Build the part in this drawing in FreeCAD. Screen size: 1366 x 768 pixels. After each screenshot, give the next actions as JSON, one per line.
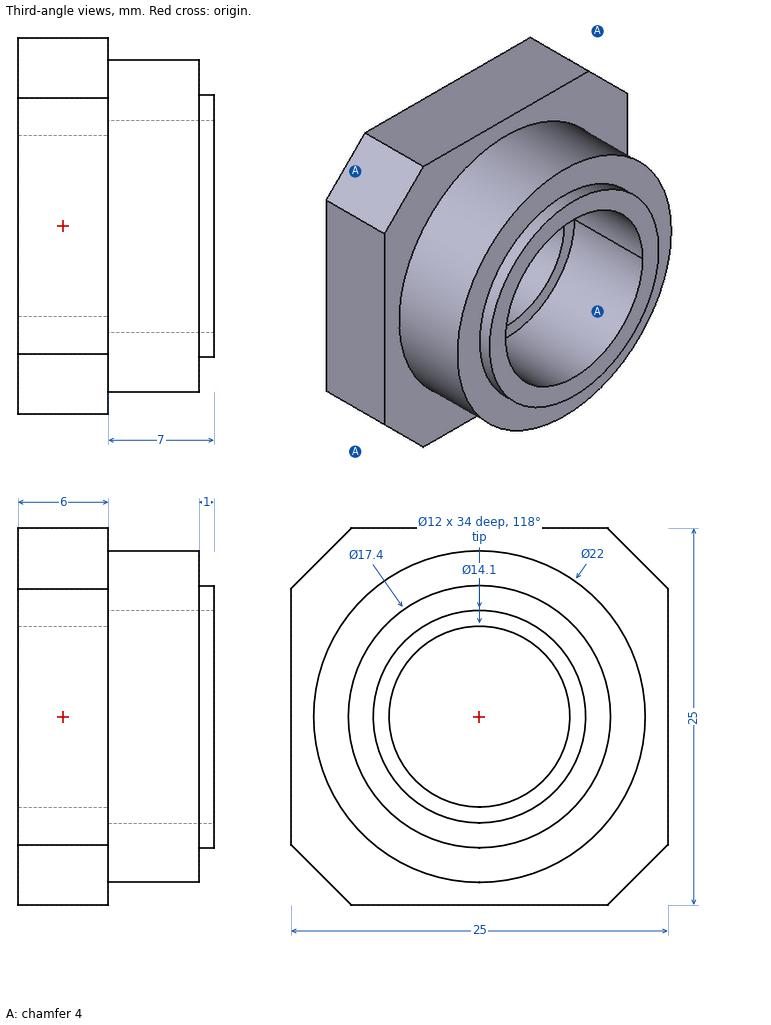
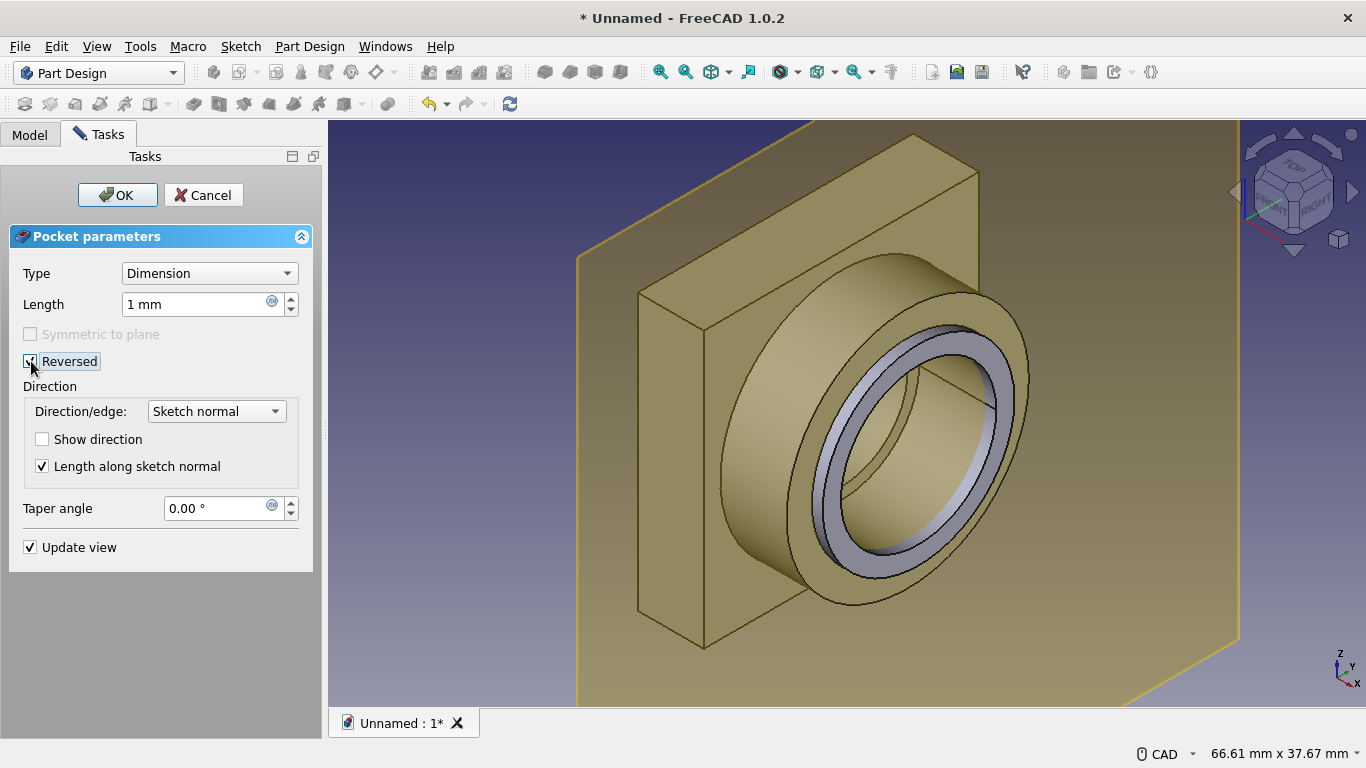
{"action": "left_click", "coordinate": [118, 195]}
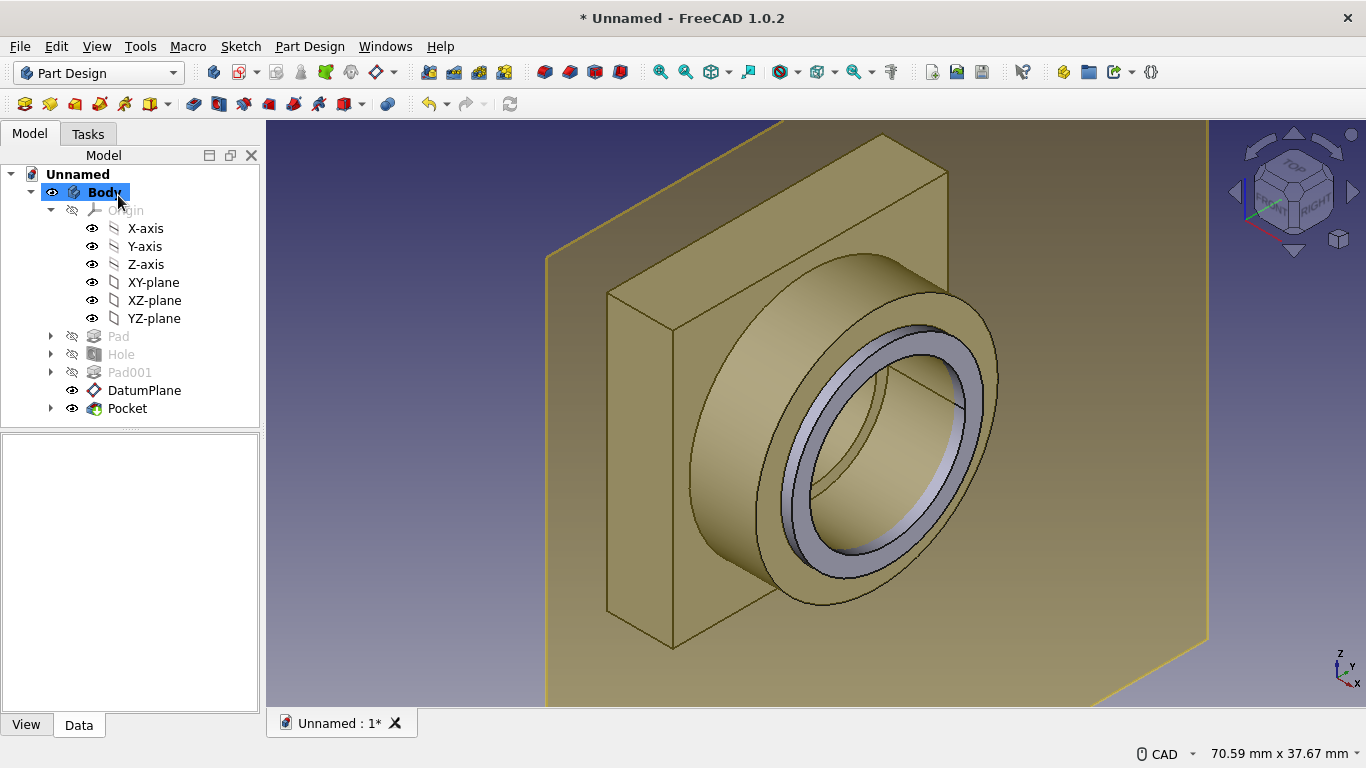
{"action": "left_click", "coordinate": [117, 390]}
{"action": "key", "text": "space"}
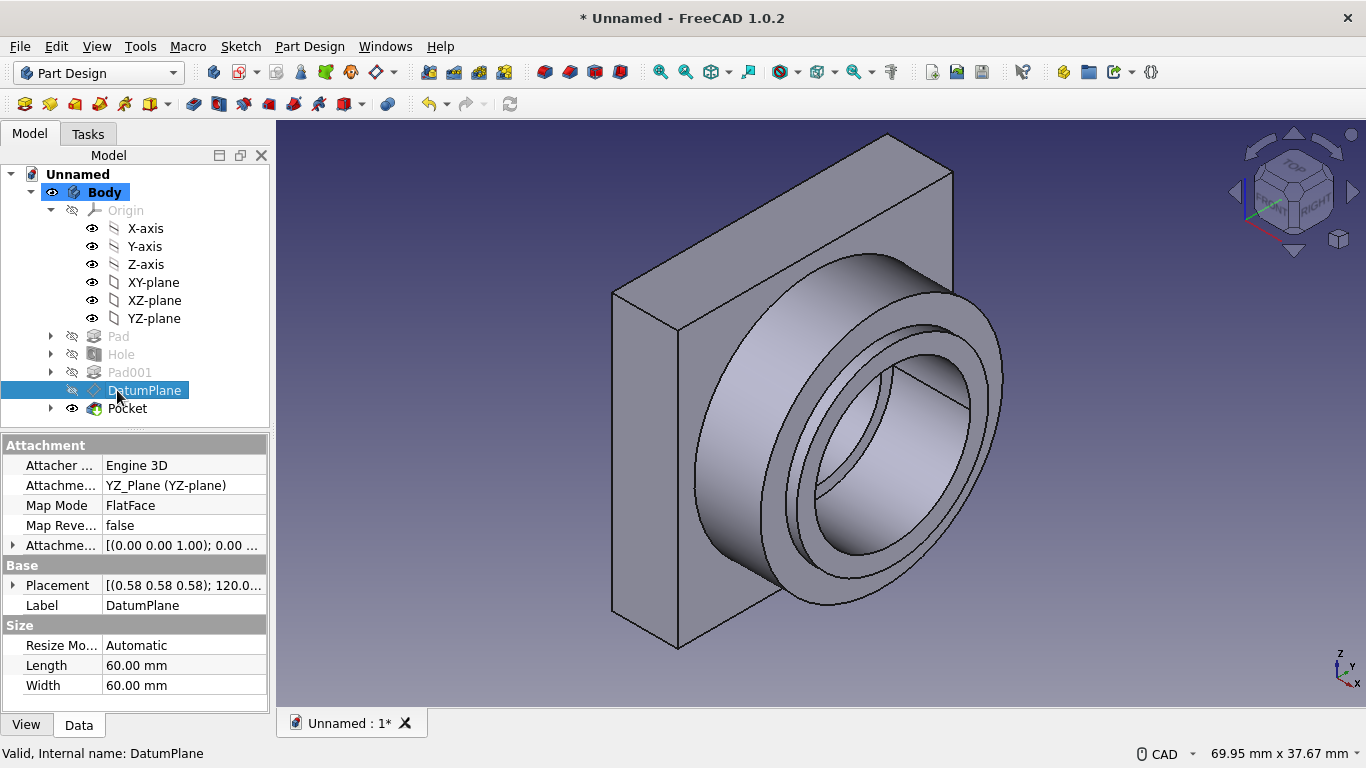
{"action": "left_click", "coordinate": [645, 311]}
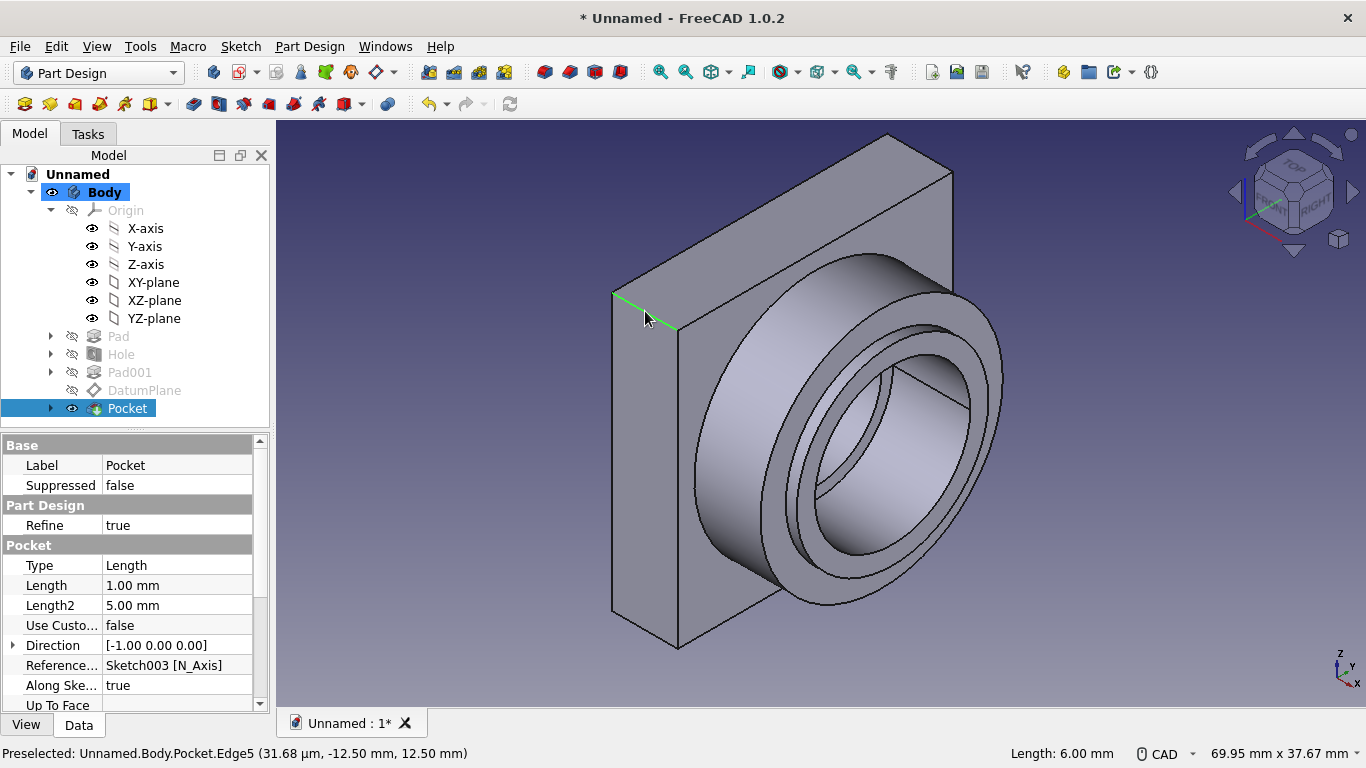
{"action": "key", "text": "2"}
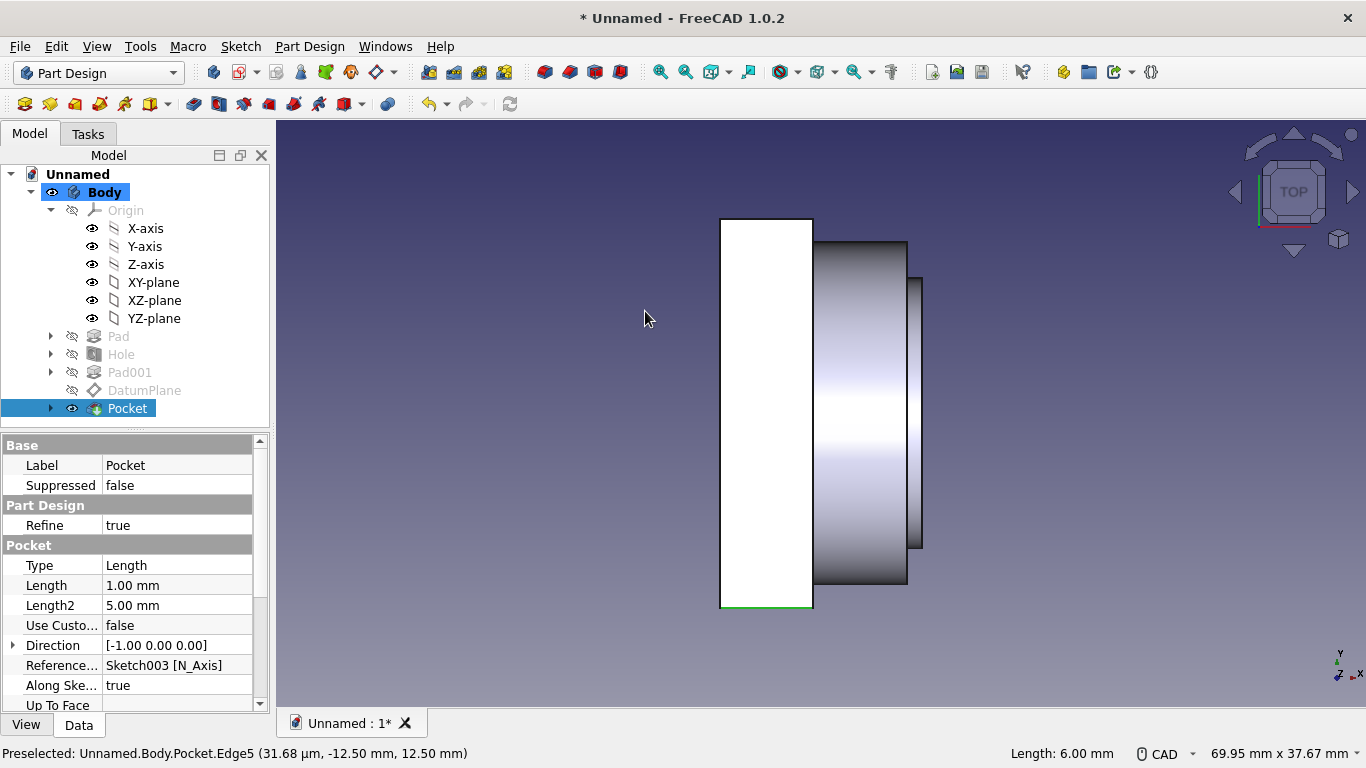
{"action": "left_click", "coordinate": [766, 218], "text": "ctrl"}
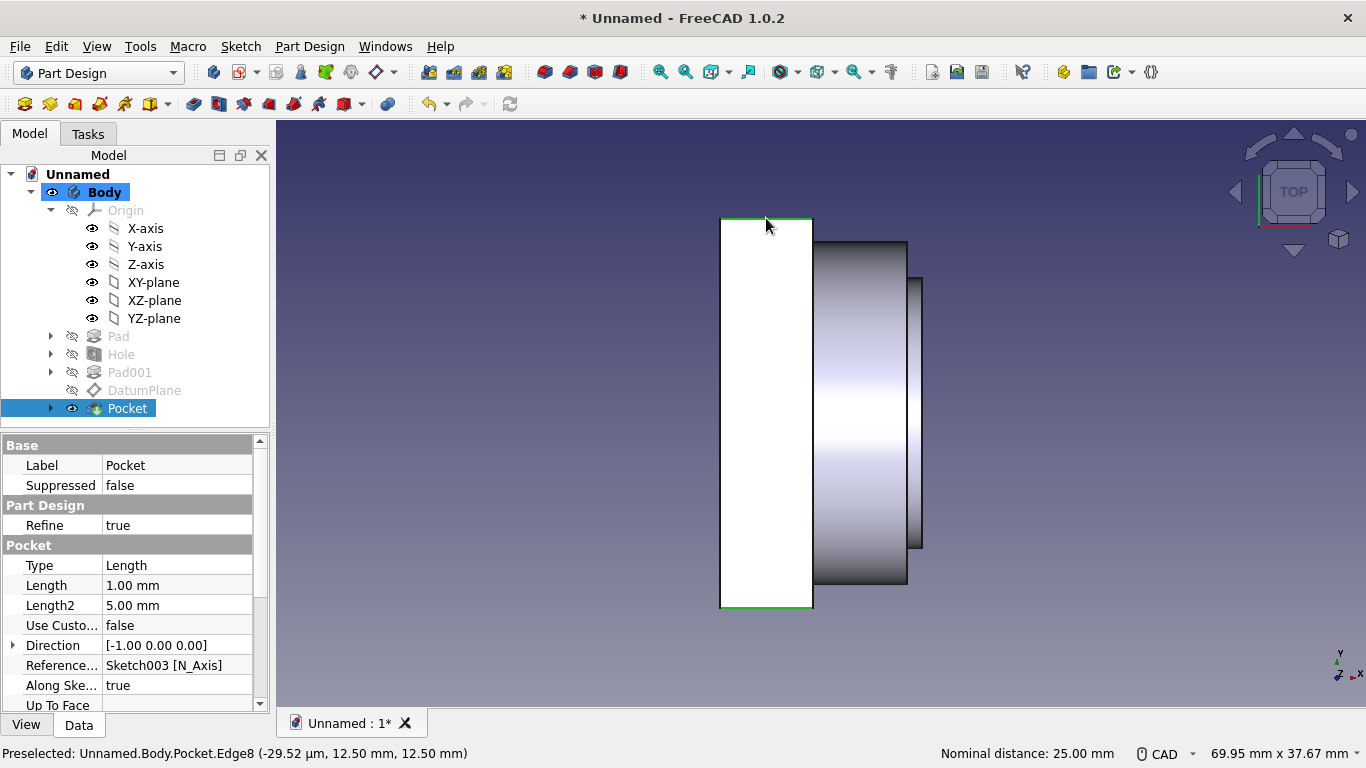
{"action": "key", "text": "0"}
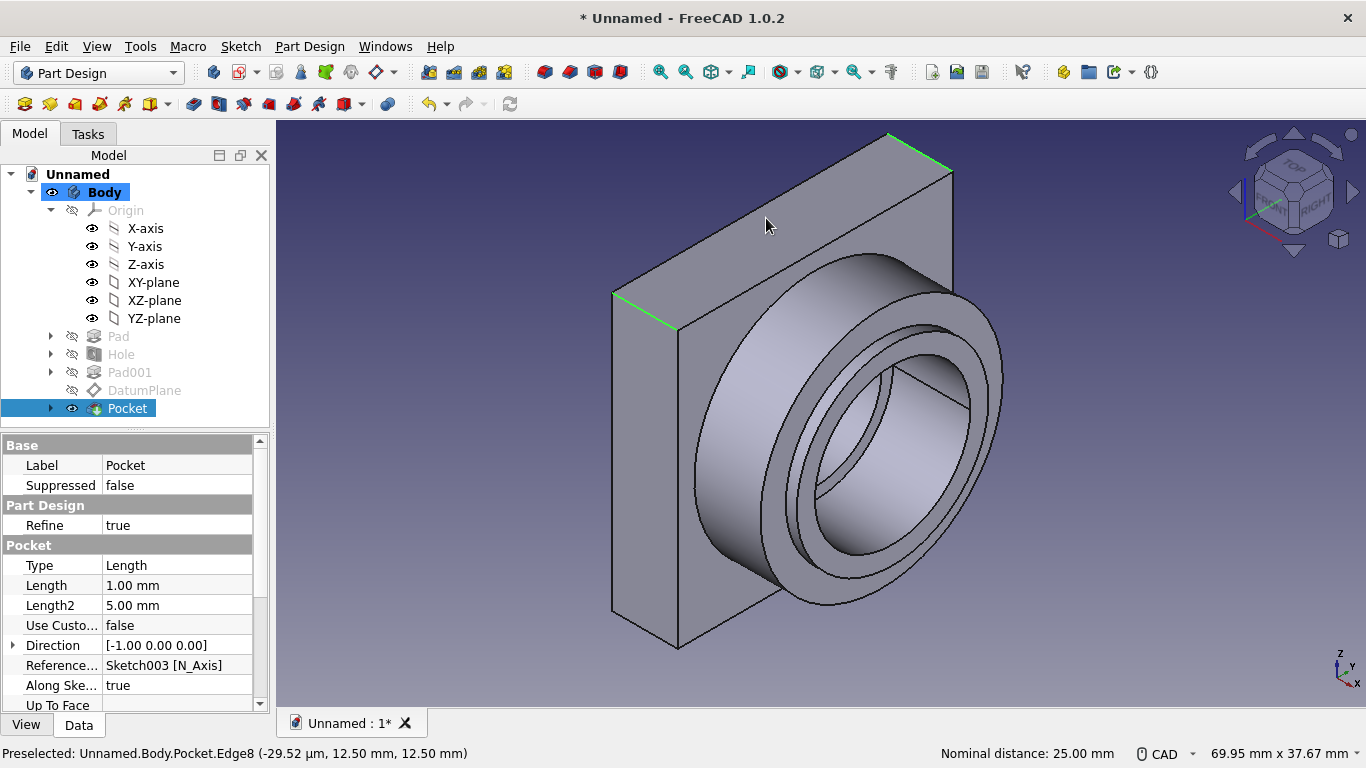
{"action": "key", "text": "1"}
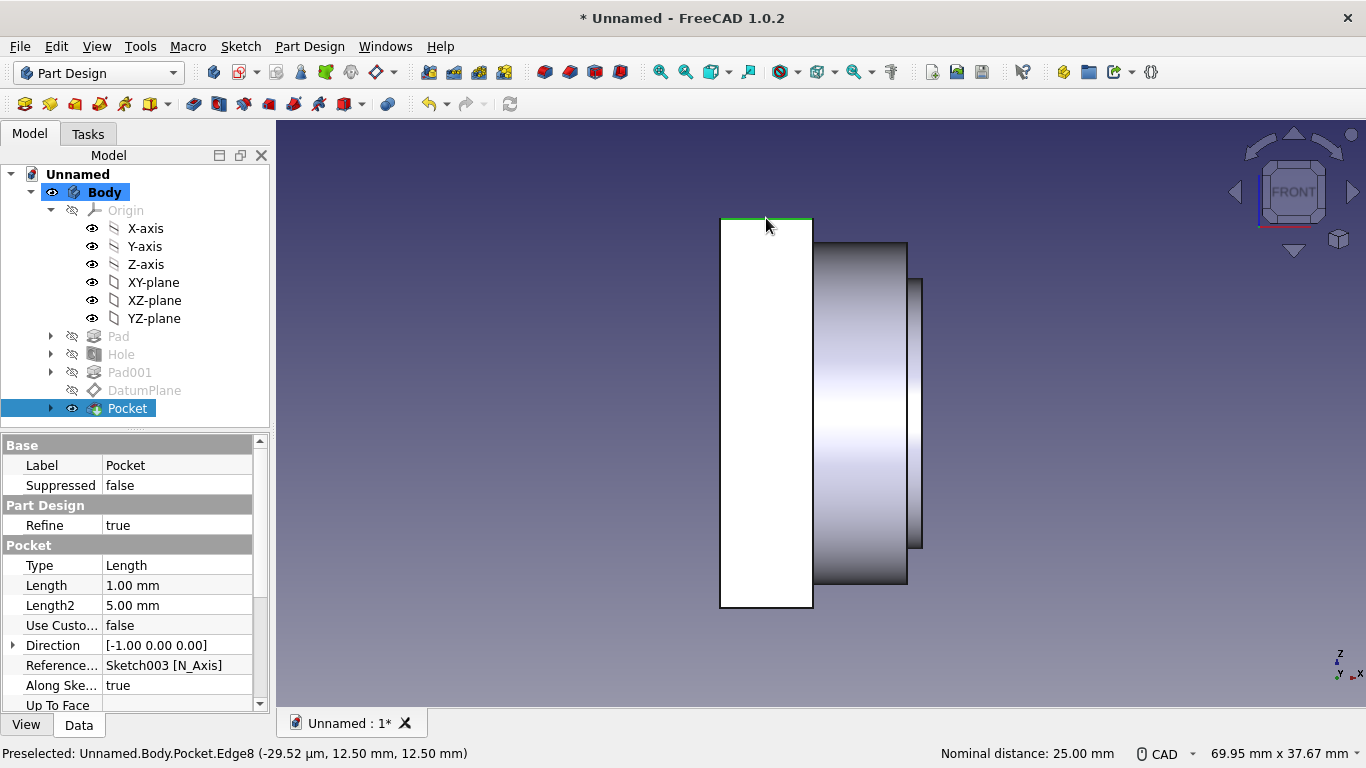
{"action": "left_click", "coordinate": [766, 607], "text": "ctrl"}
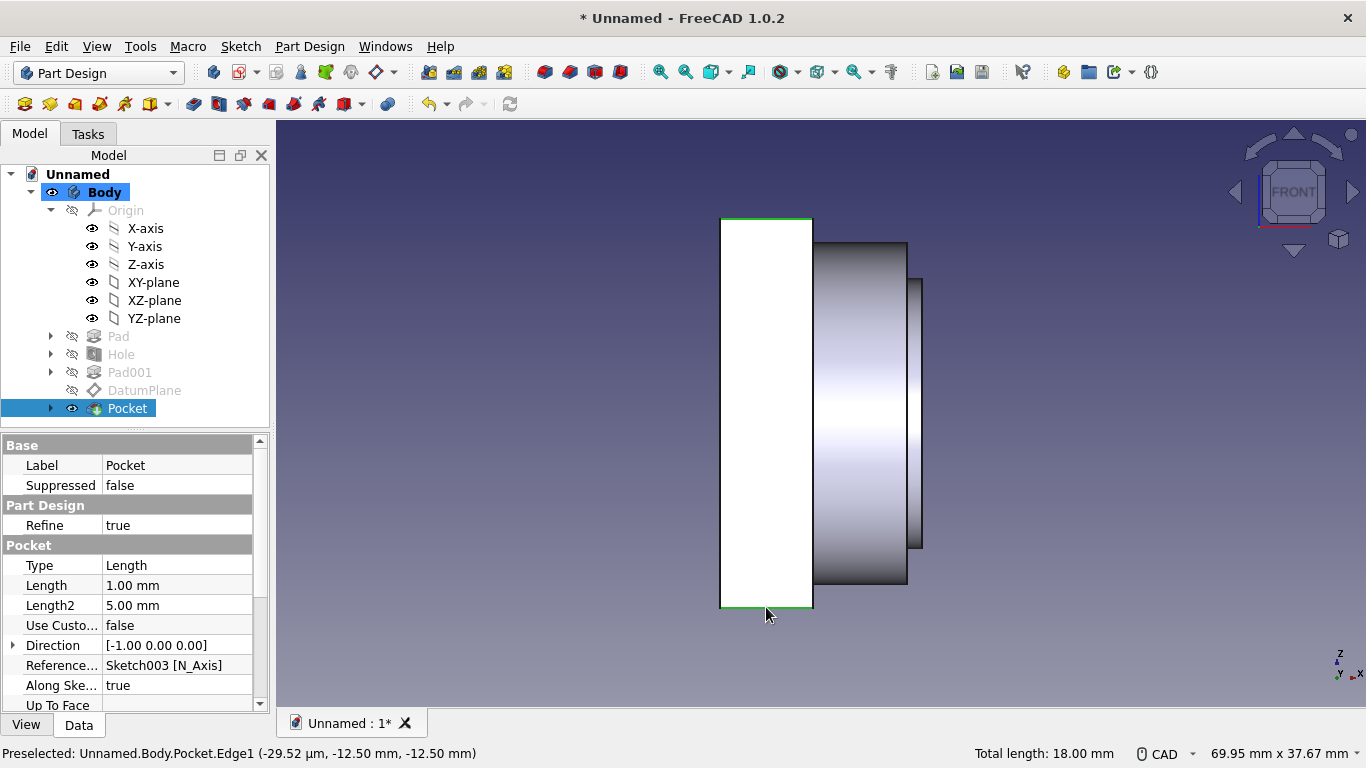
{"action": "key", "text": "3"}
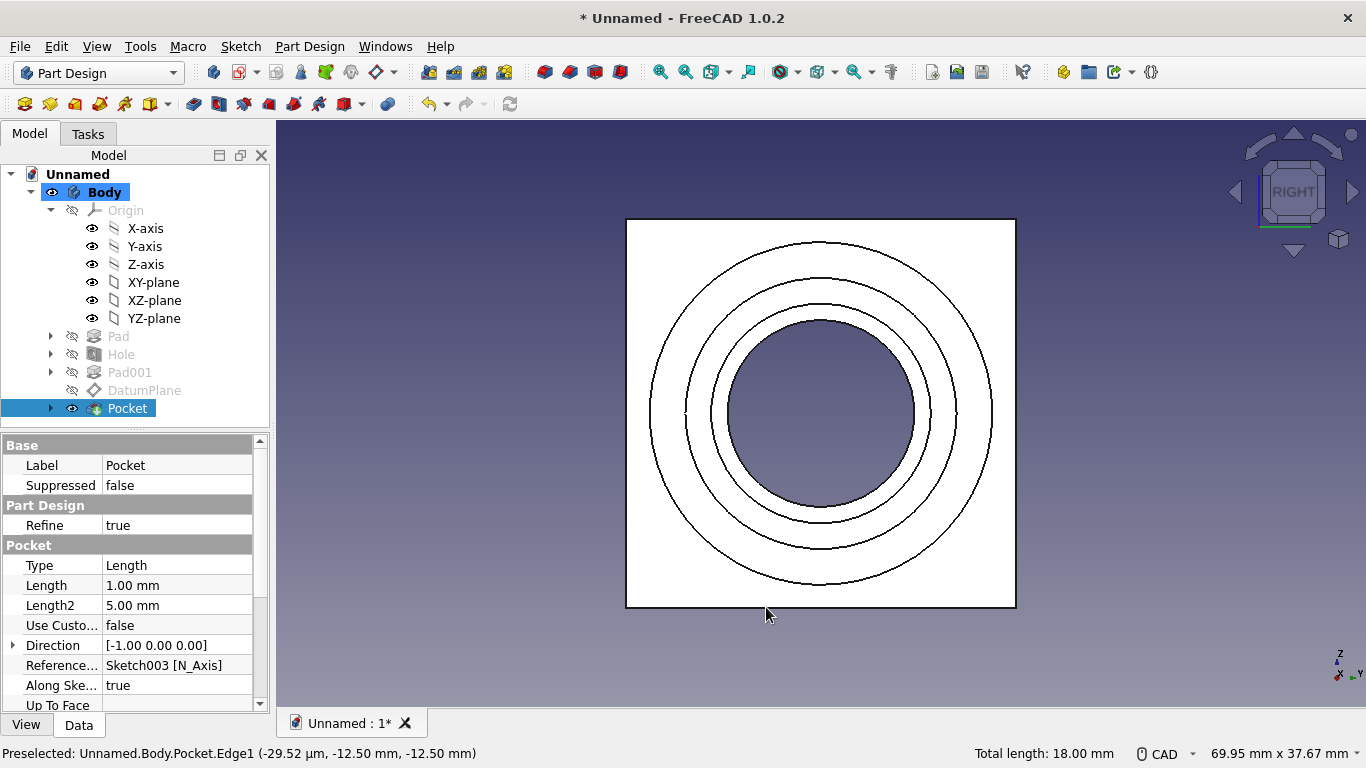
{"action": "key", "text": "5"}